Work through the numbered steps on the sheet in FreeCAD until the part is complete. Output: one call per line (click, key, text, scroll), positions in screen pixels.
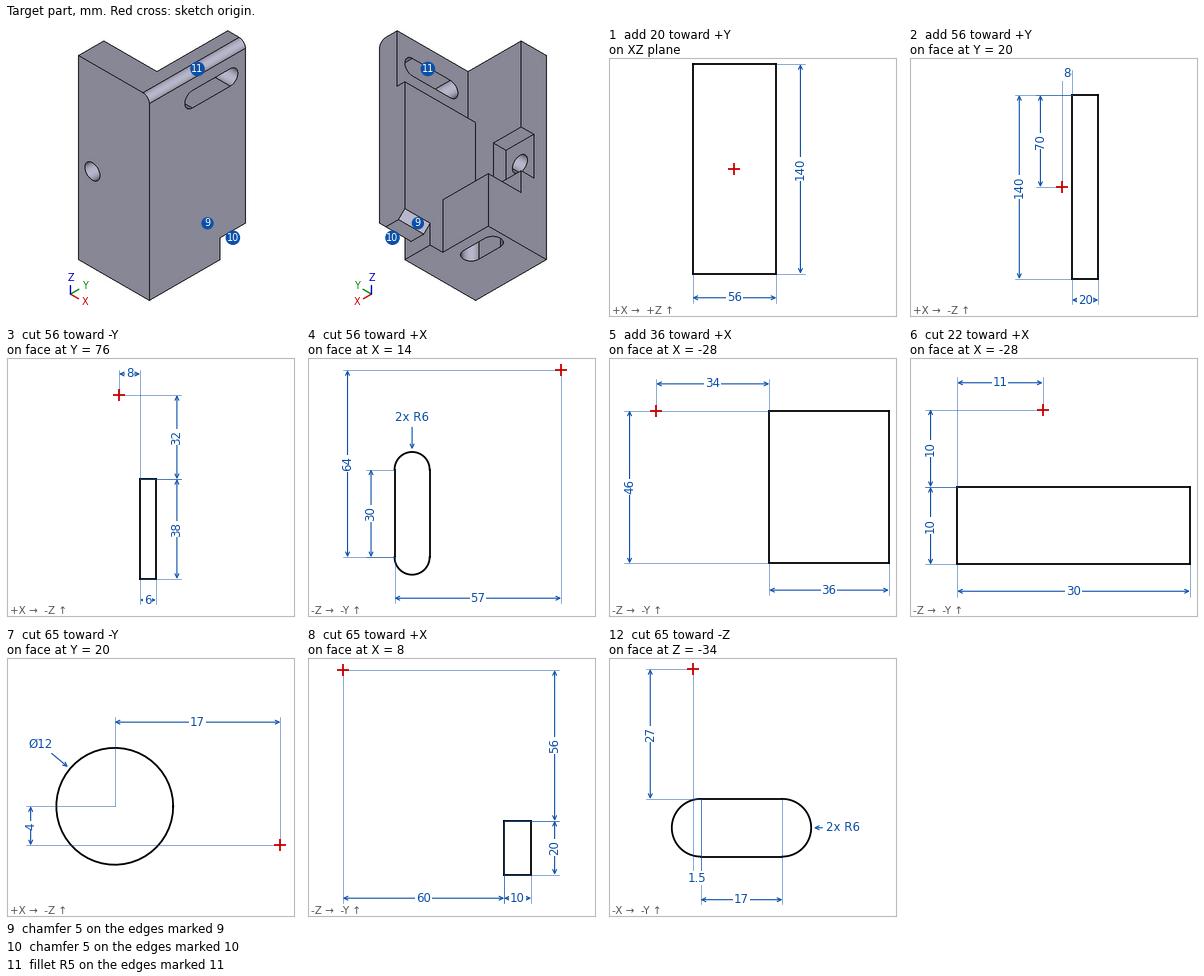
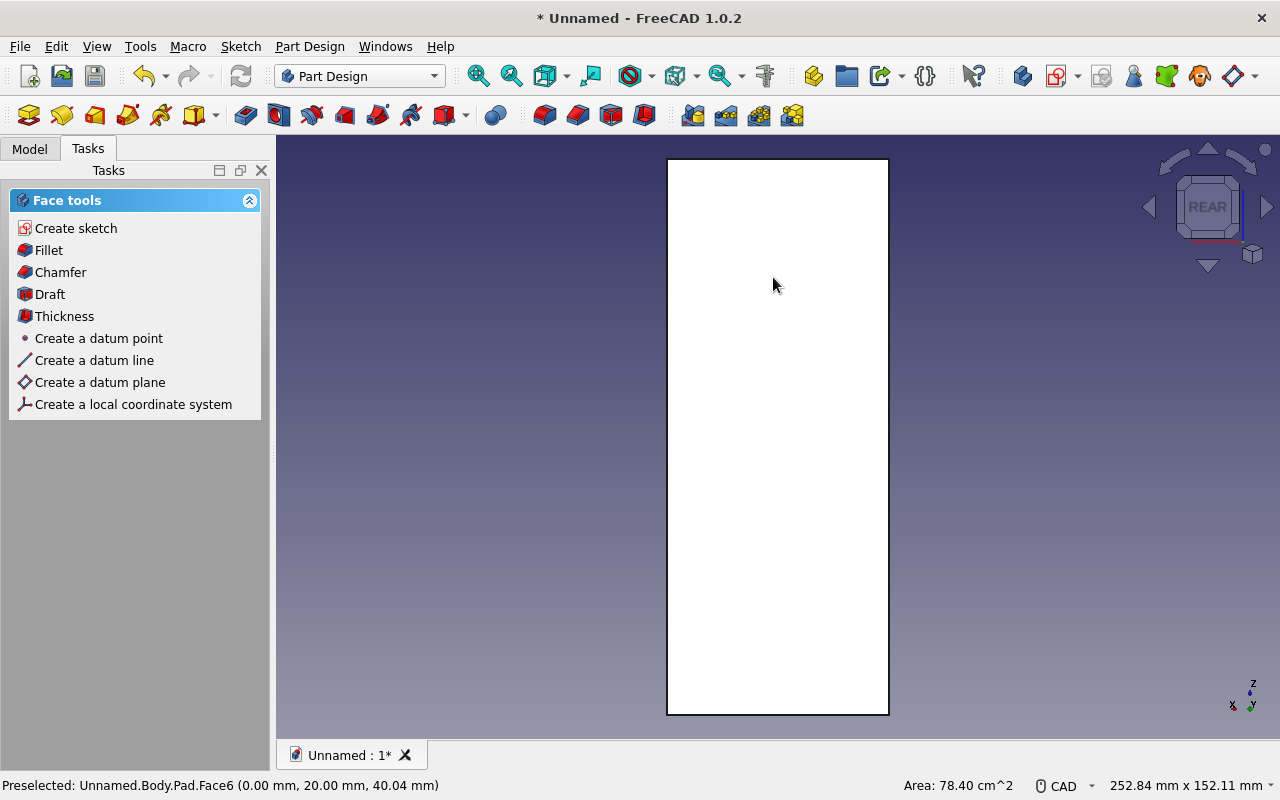
click(1056, 76)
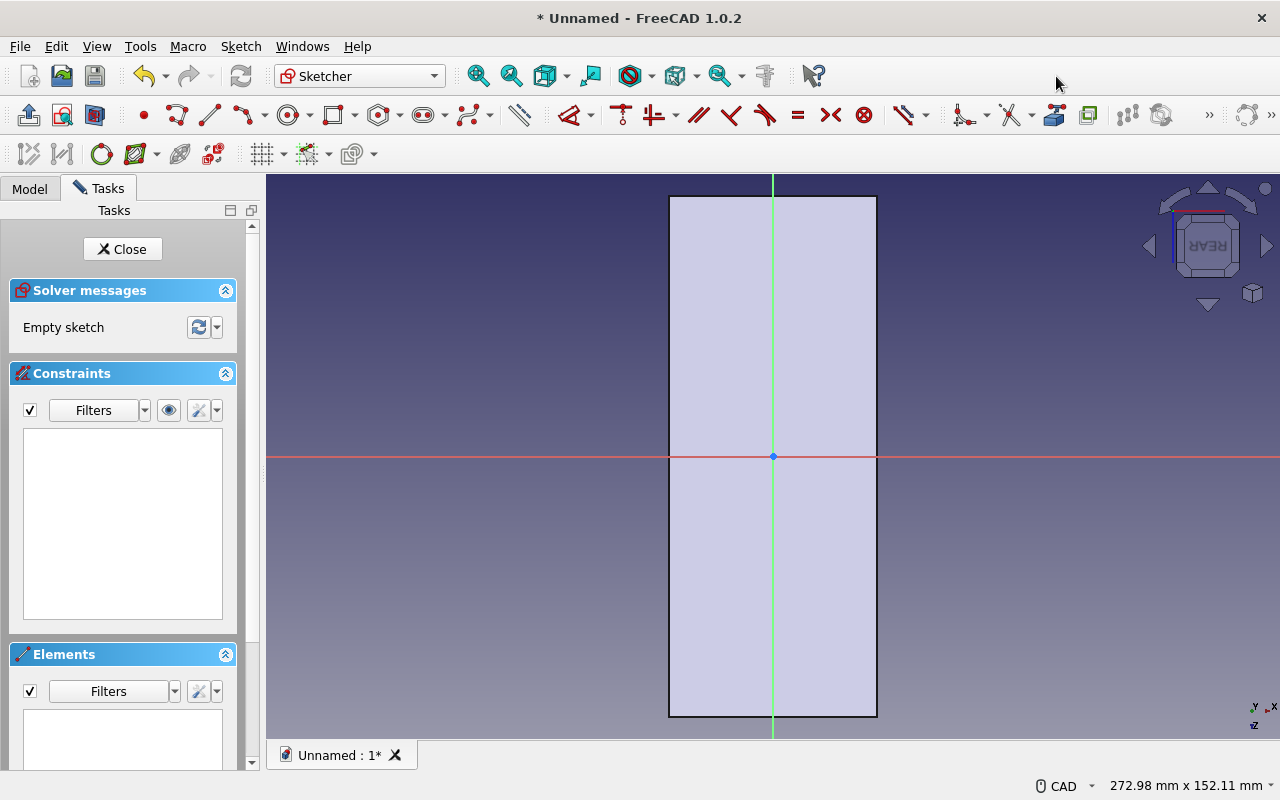
scroll(459, 457, down, 2)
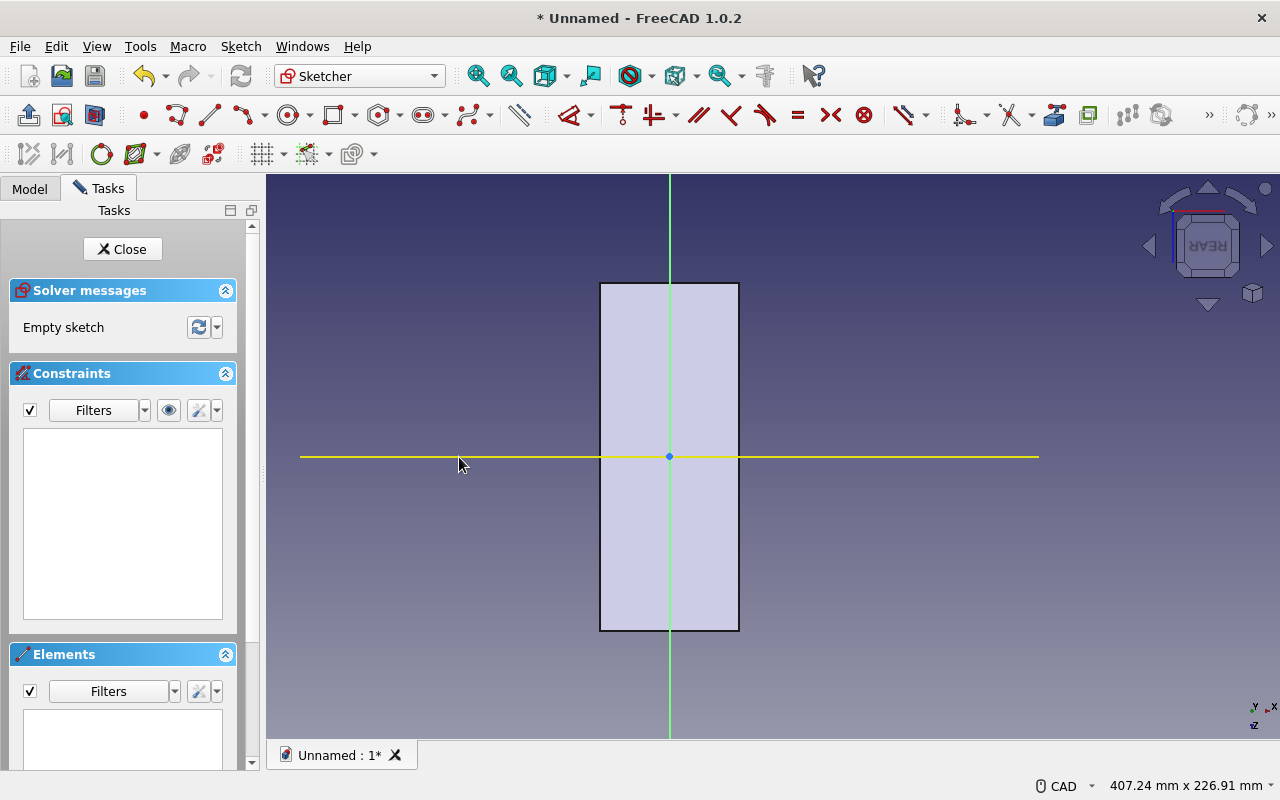
click(332, 116)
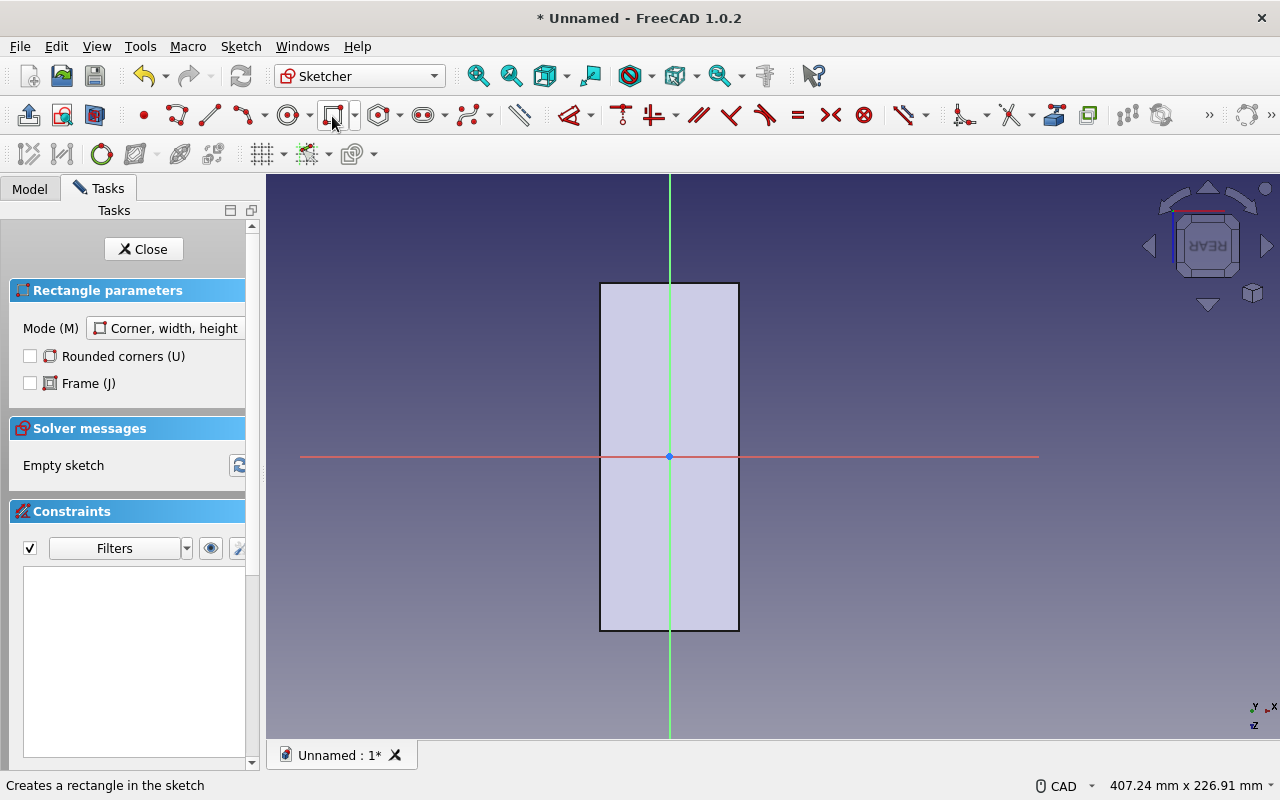
click(689, 283)
click(739, 631)
key(Escape)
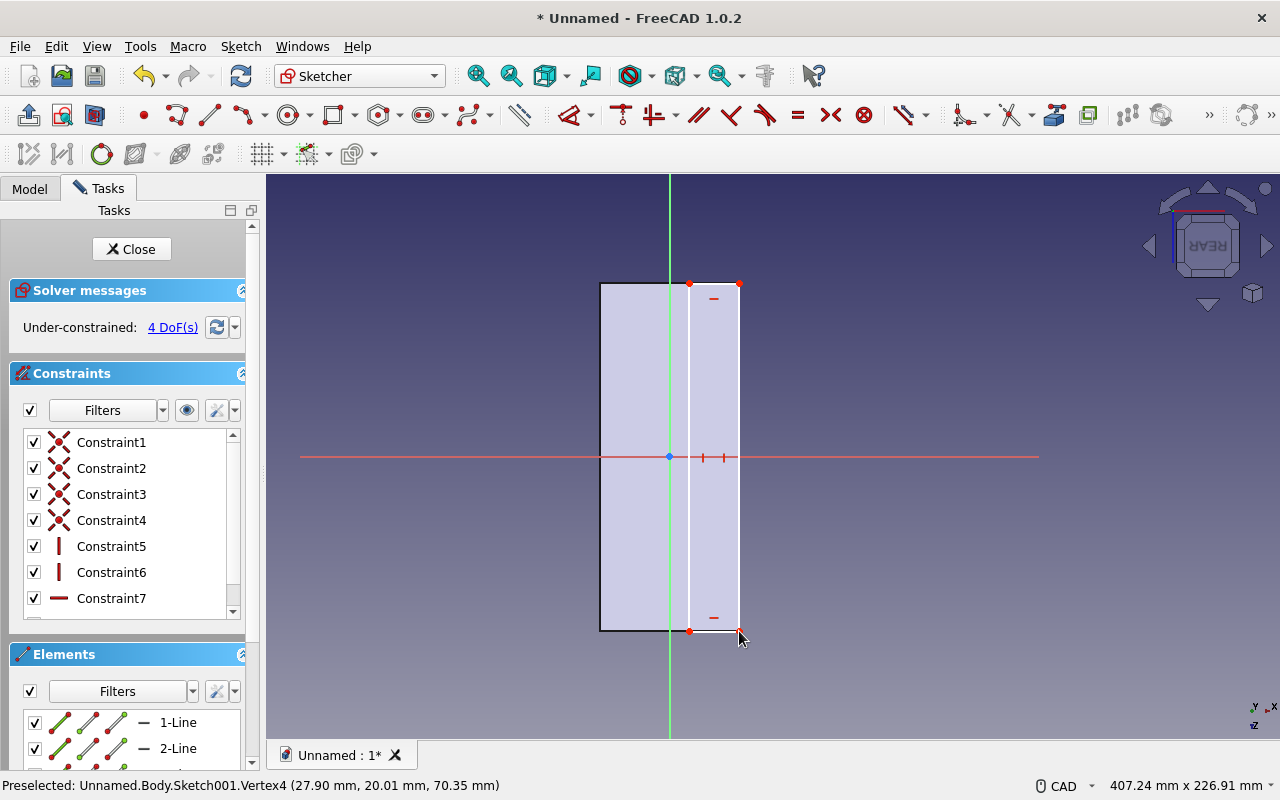
click(568, 116)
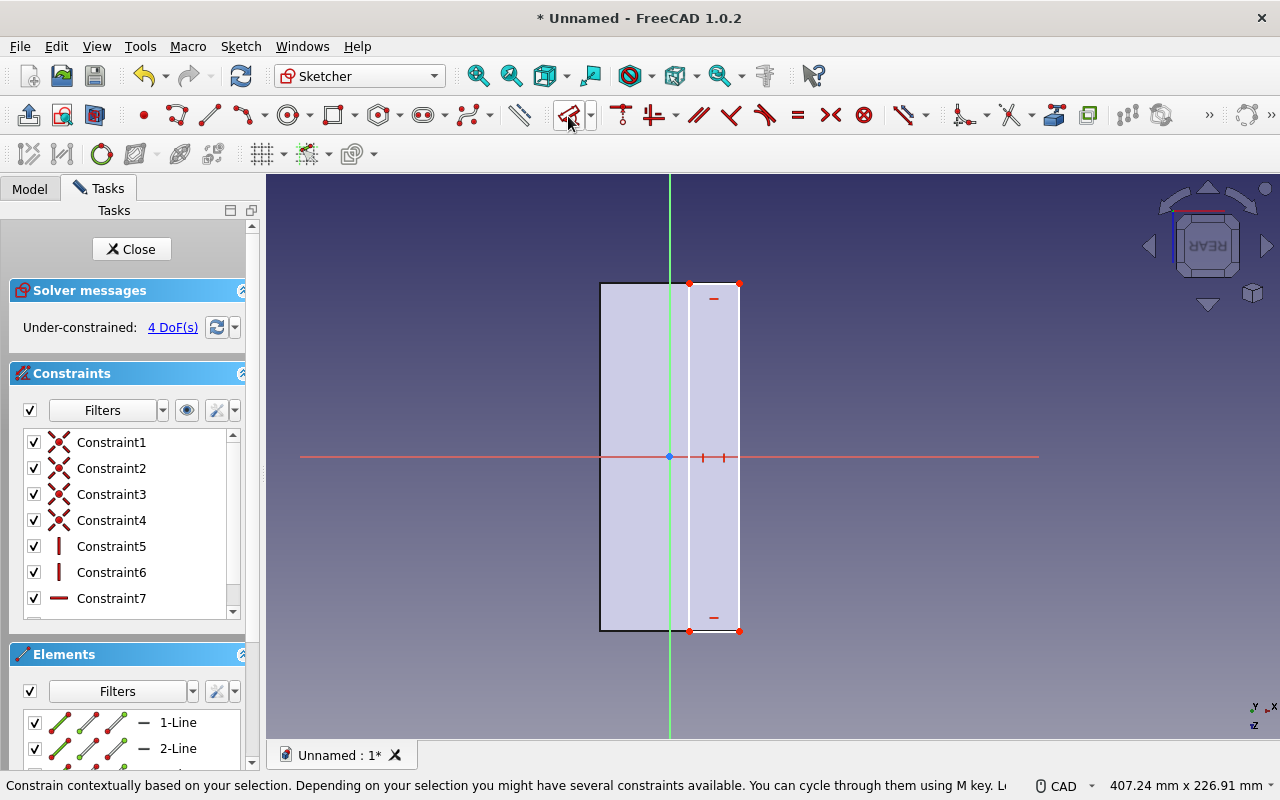
click(704, 632)
click(714, 666)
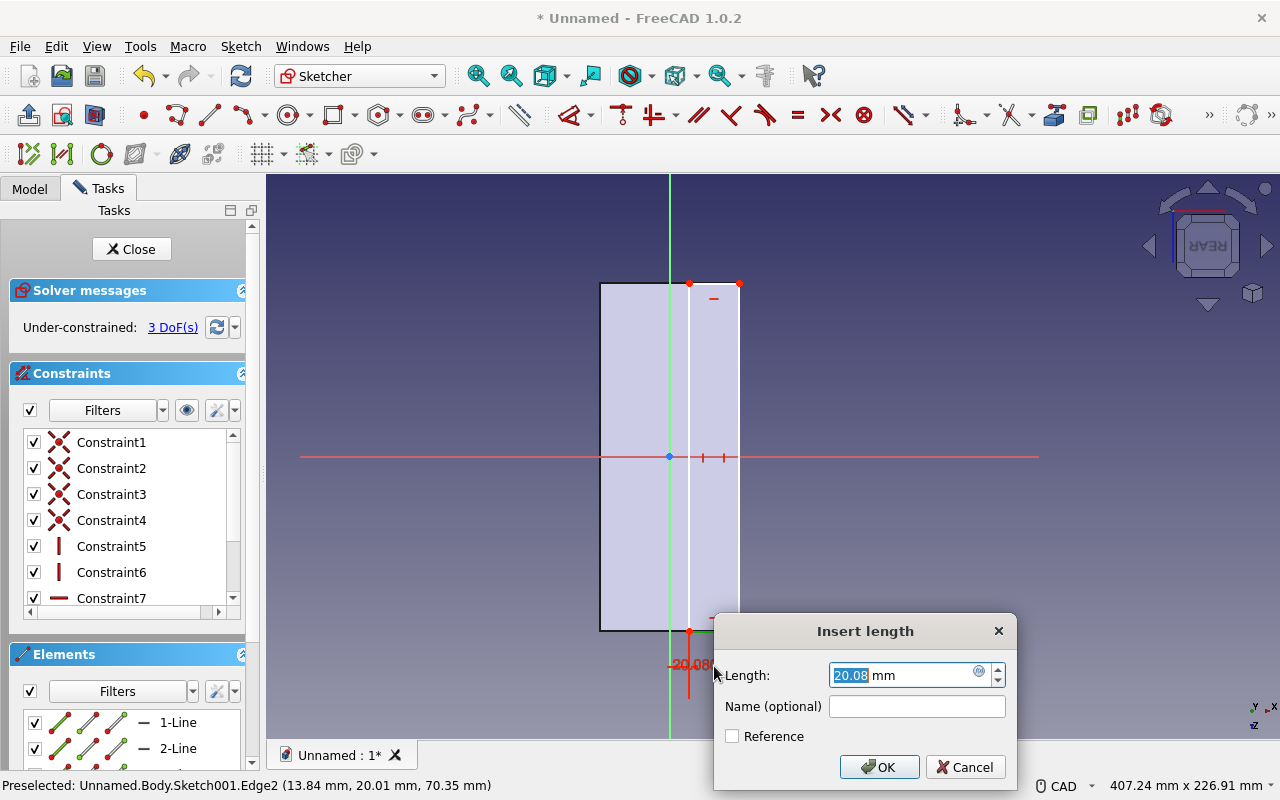
text(20)
key(Return)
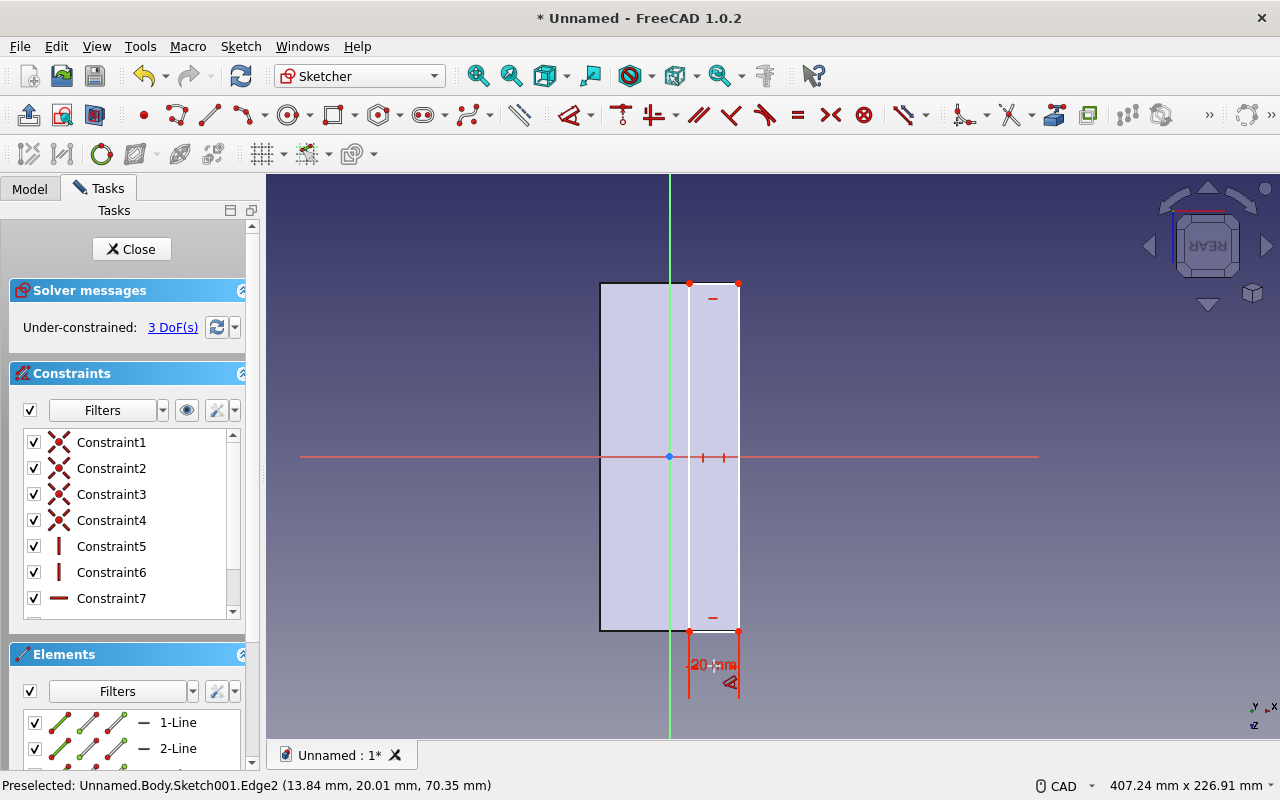
scroll(689, 284, up, 4)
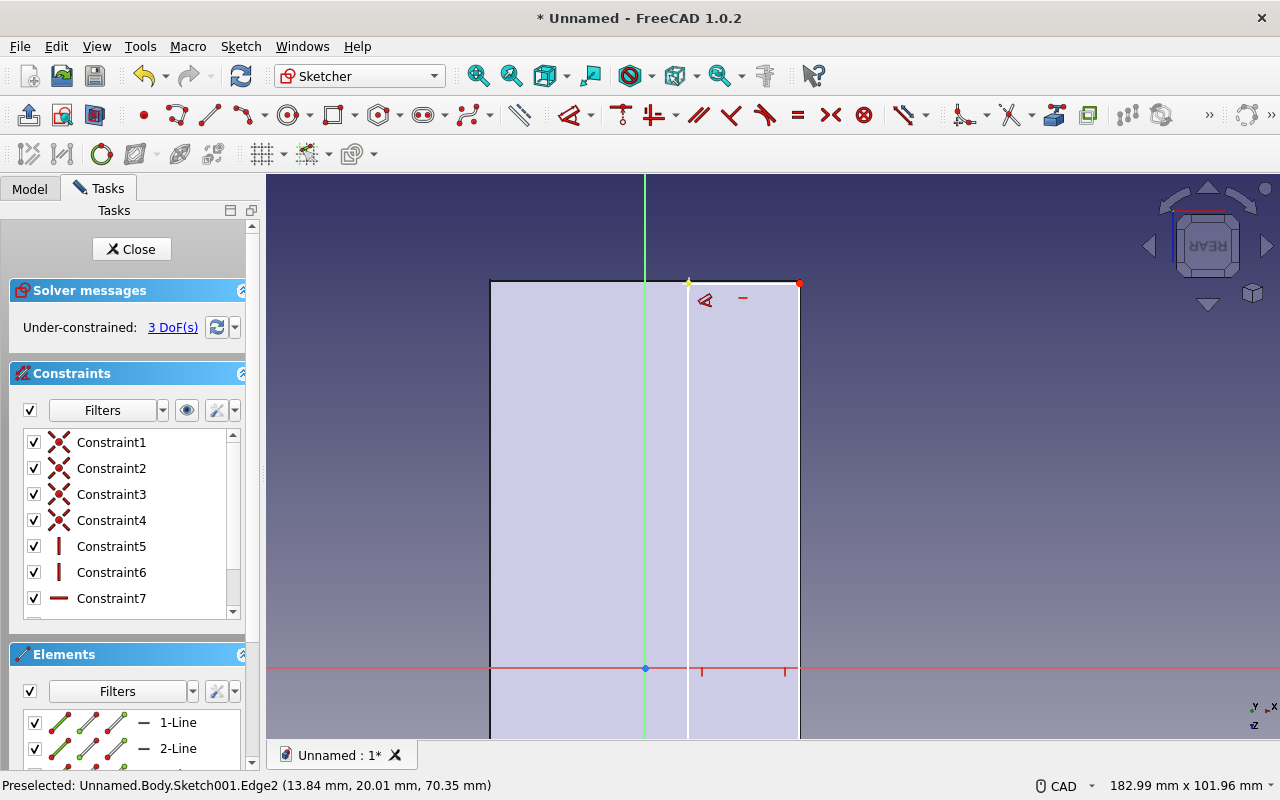
click(688, 284)
click(667, 250)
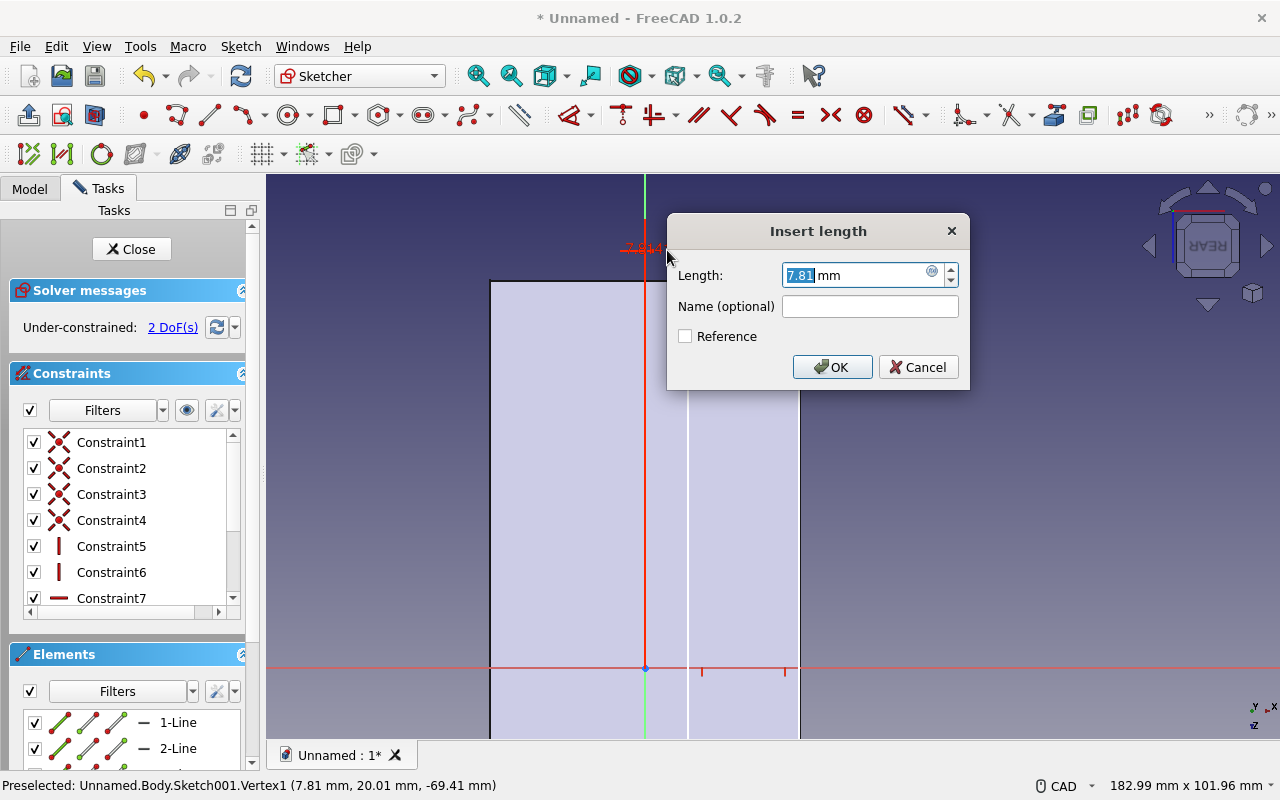
text(8)
key(Return)